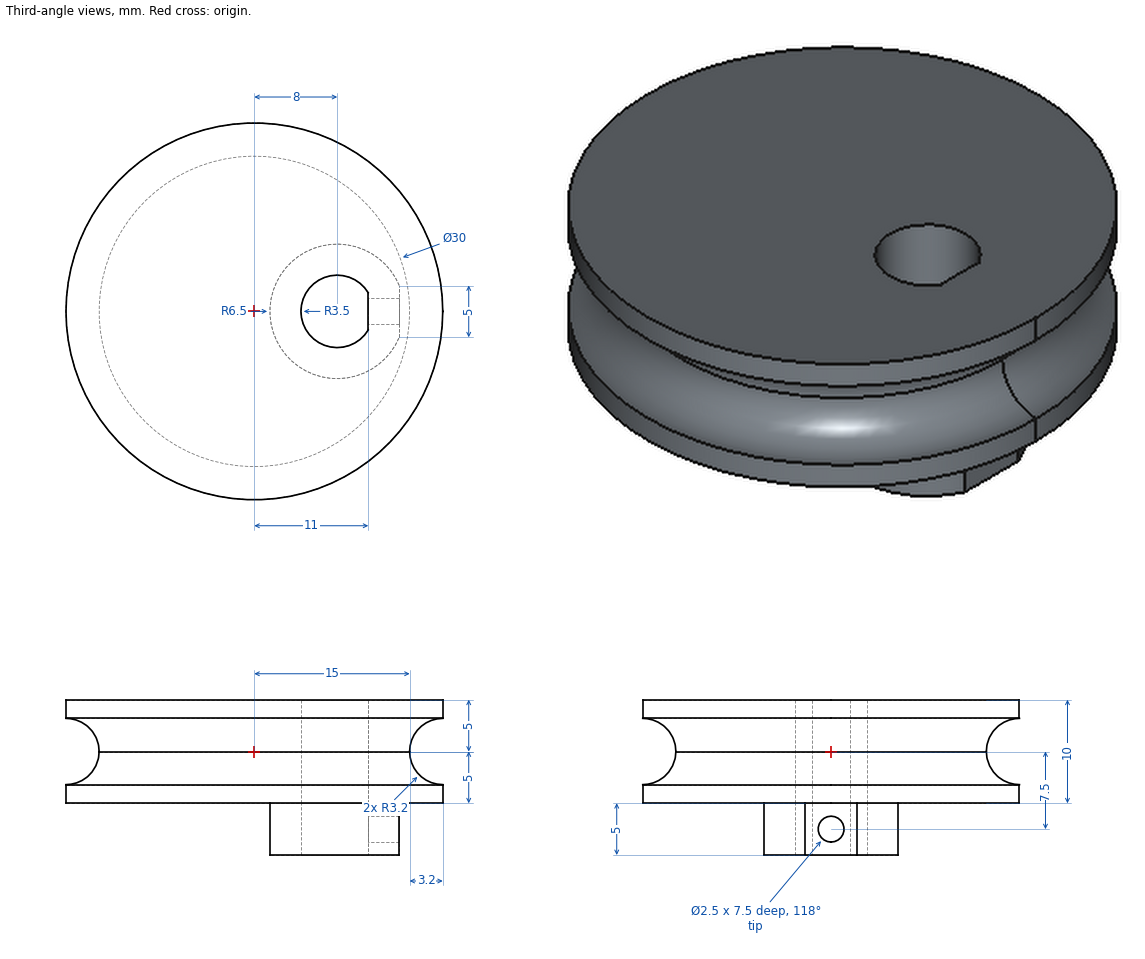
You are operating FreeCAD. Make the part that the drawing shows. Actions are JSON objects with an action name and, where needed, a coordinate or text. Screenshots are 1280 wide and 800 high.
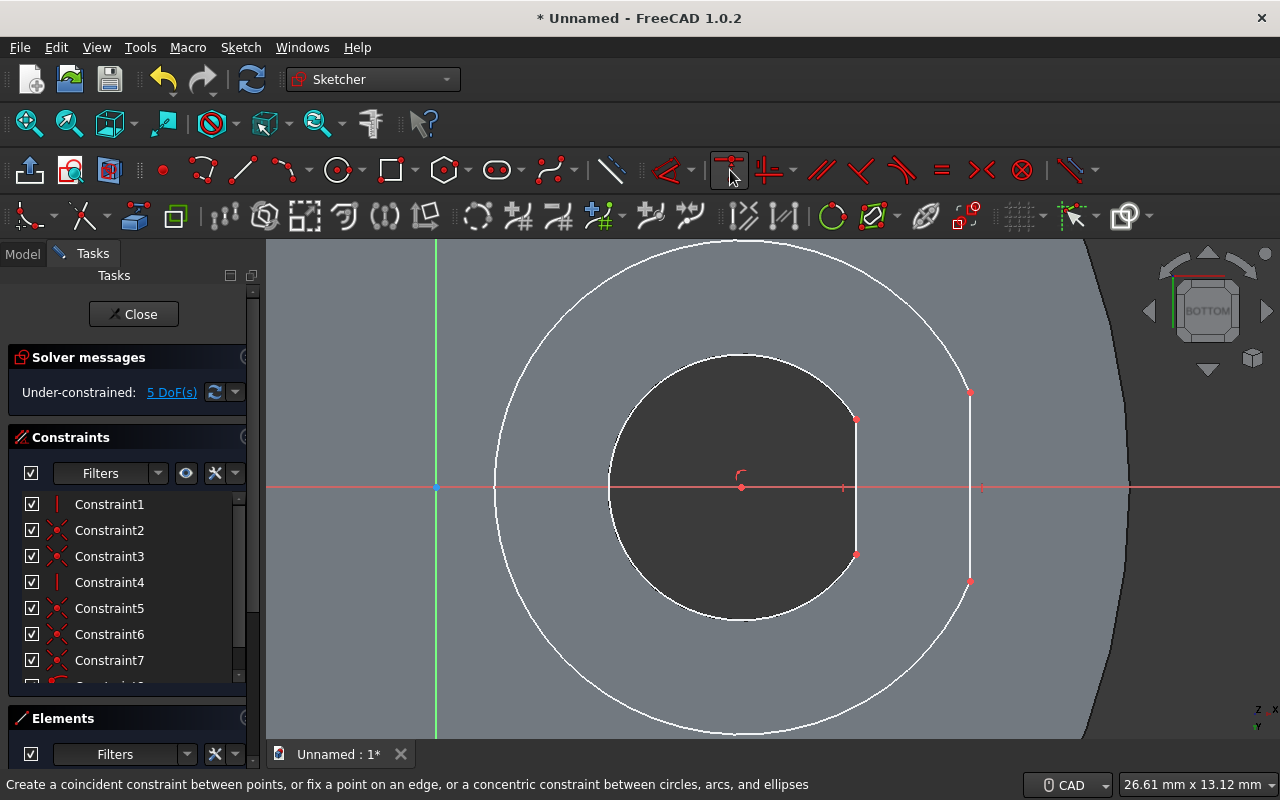
{"action": "left_click", "coordinate": [666, 170]}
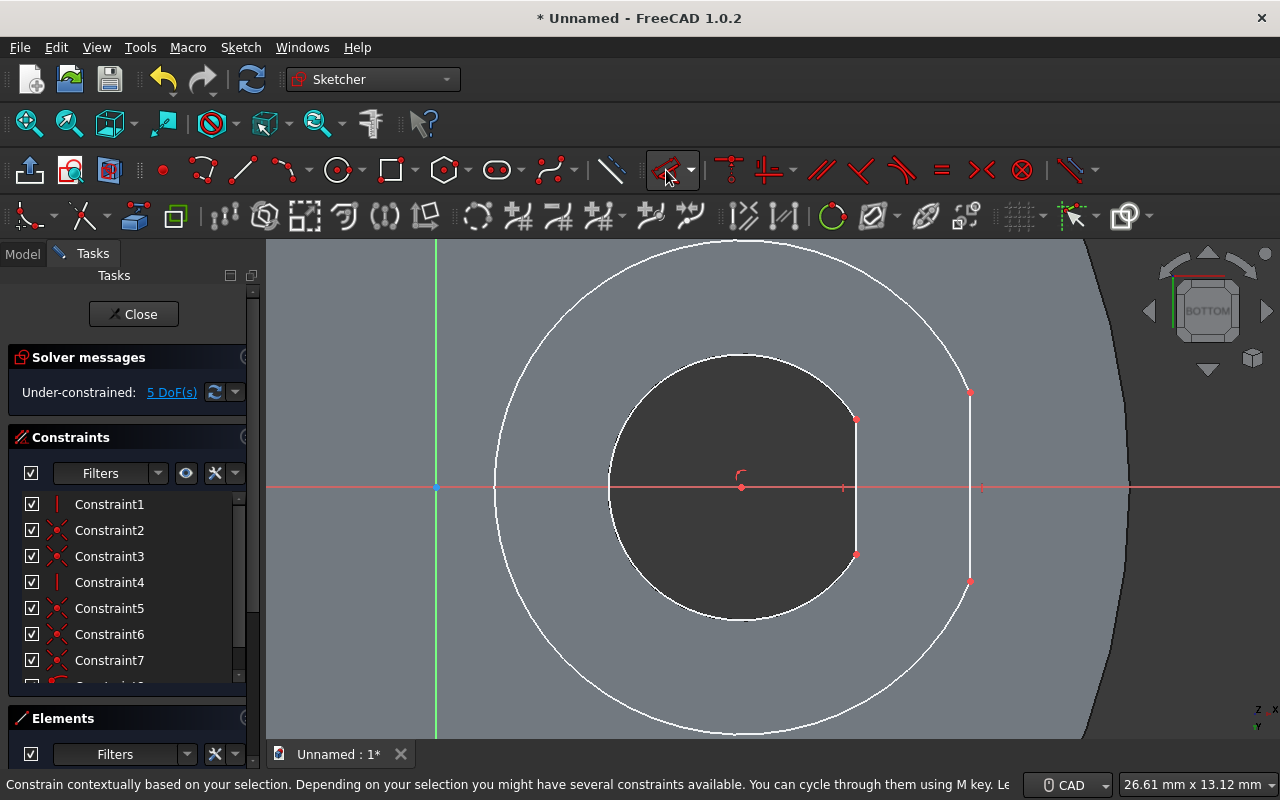
{"action": "left_click", "coordinate": [629, 267]}
{"action": "left_click", "coordinate": [511, 330]}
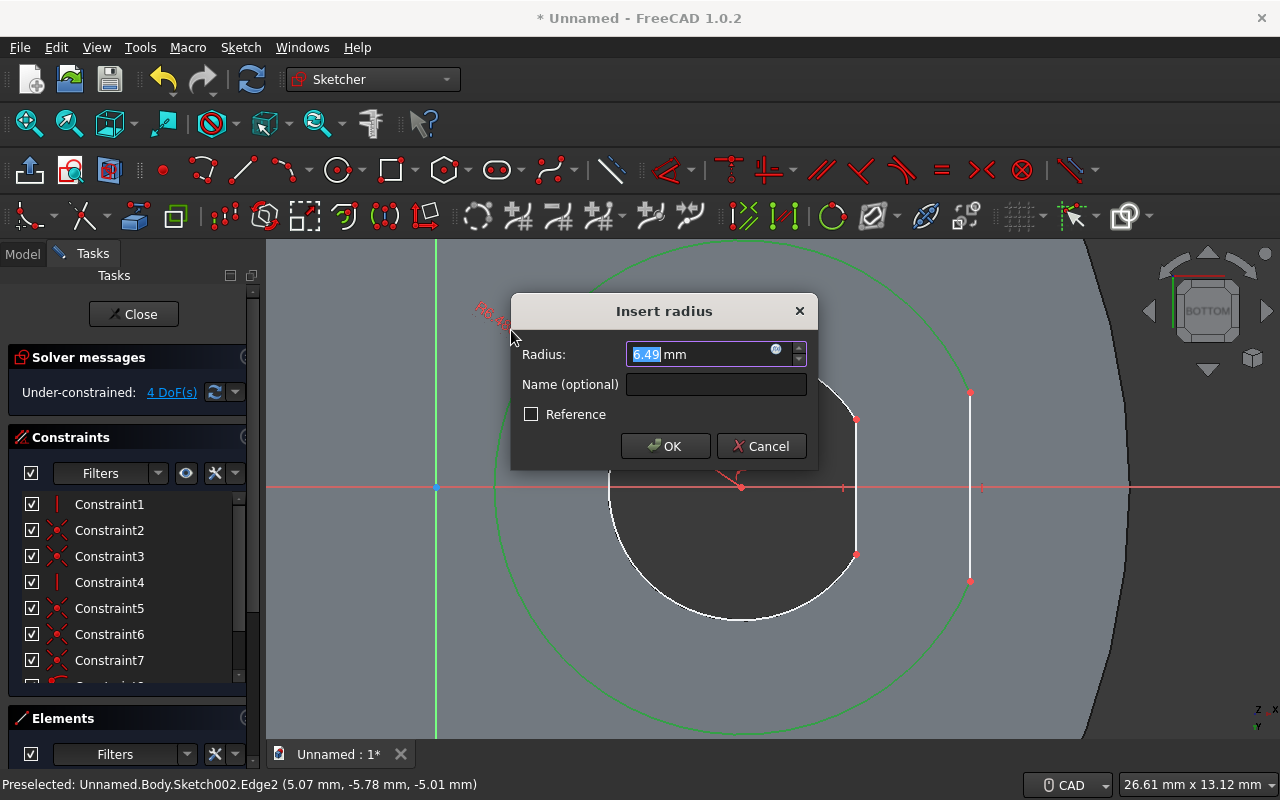
{"action": "type", "text": "6.5"}
{"action": "key", "text": "Return"}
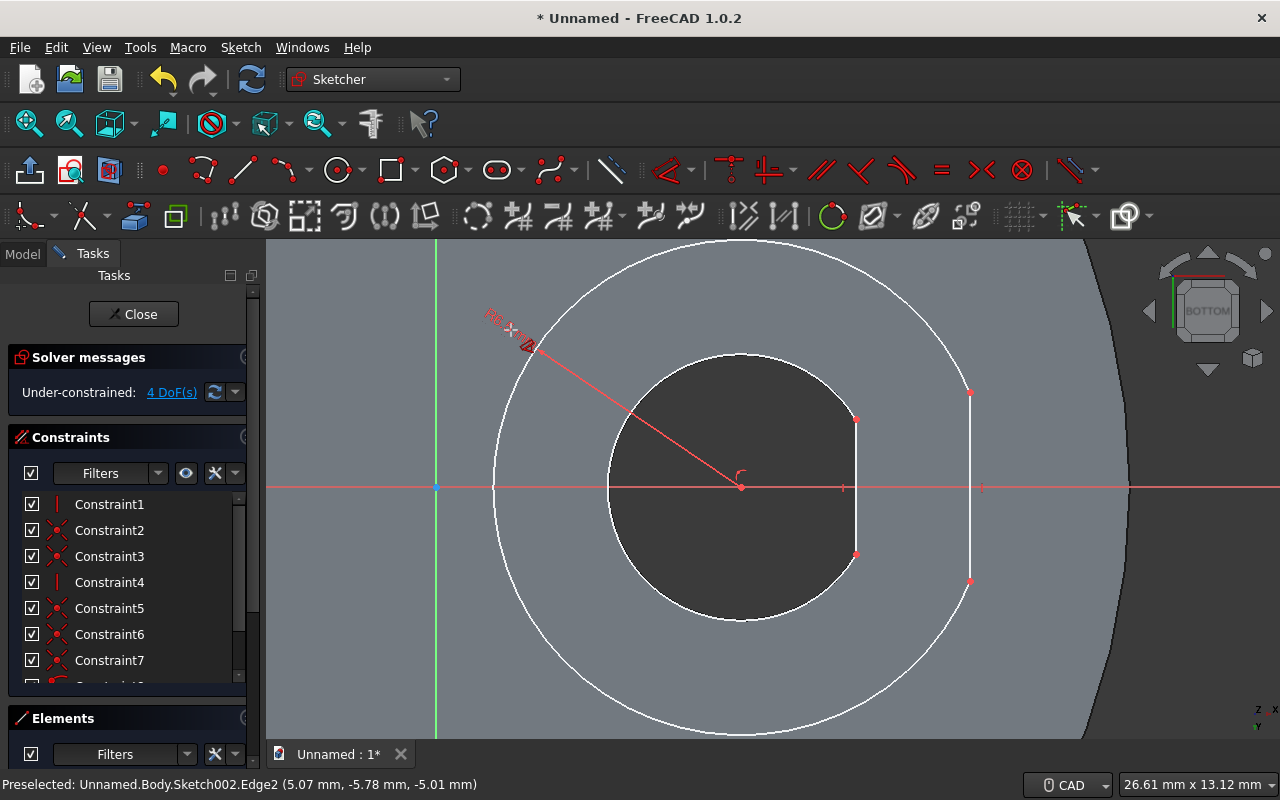
{"action": "left_click", "coordinate": [674, 372]}
{"action": "left_click", "coordinate": [658, 344]}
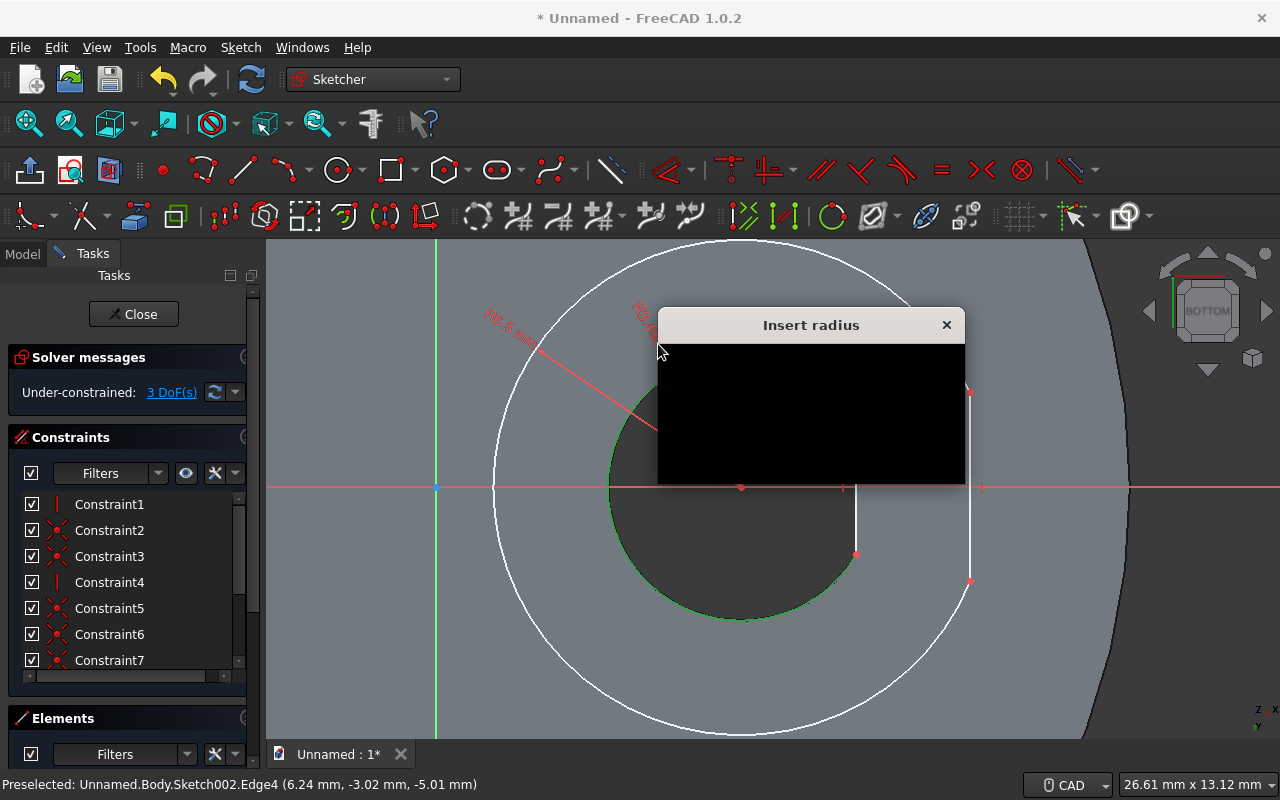
{"action": "type", "text": "3.5"}
{"action": "key", "text": "Return"}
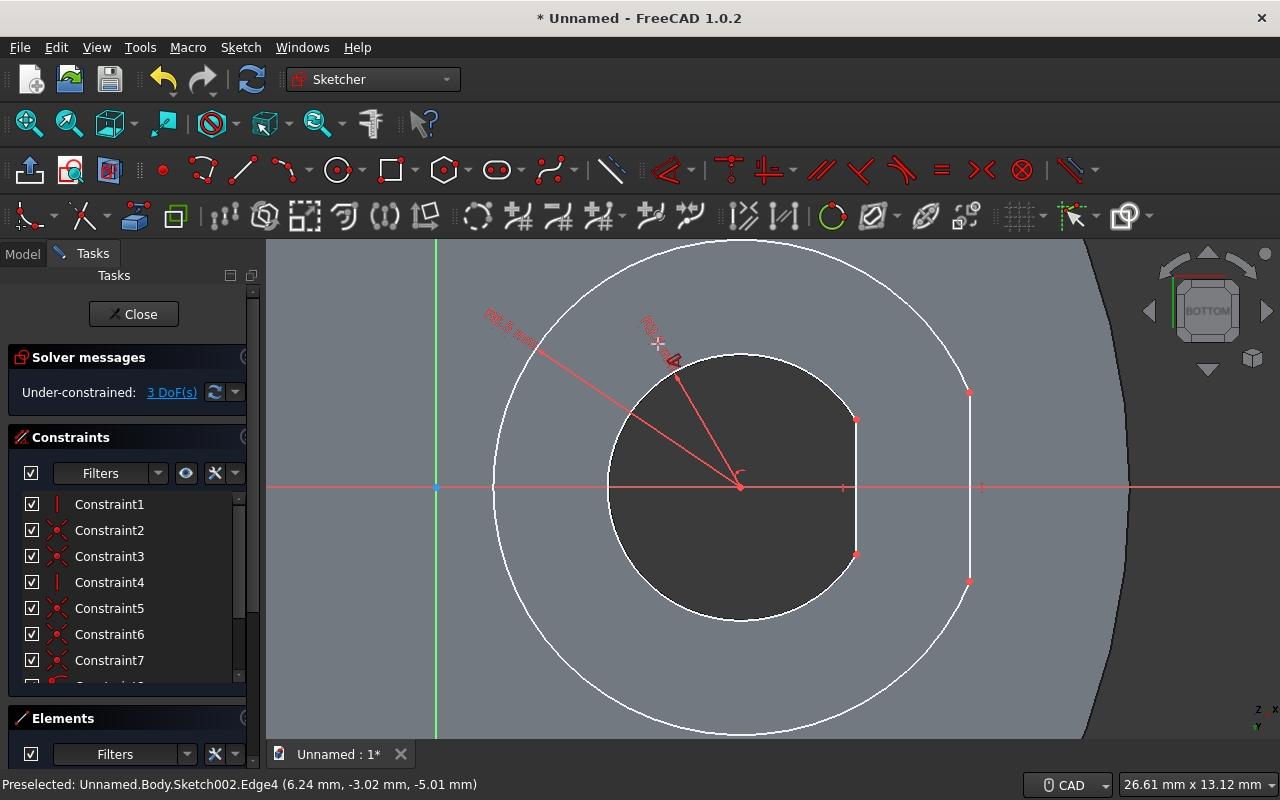
{"action": "left_click", "coordinate": [970, 450]}
{"action": "left_click", "coordinate": [1004, 444]}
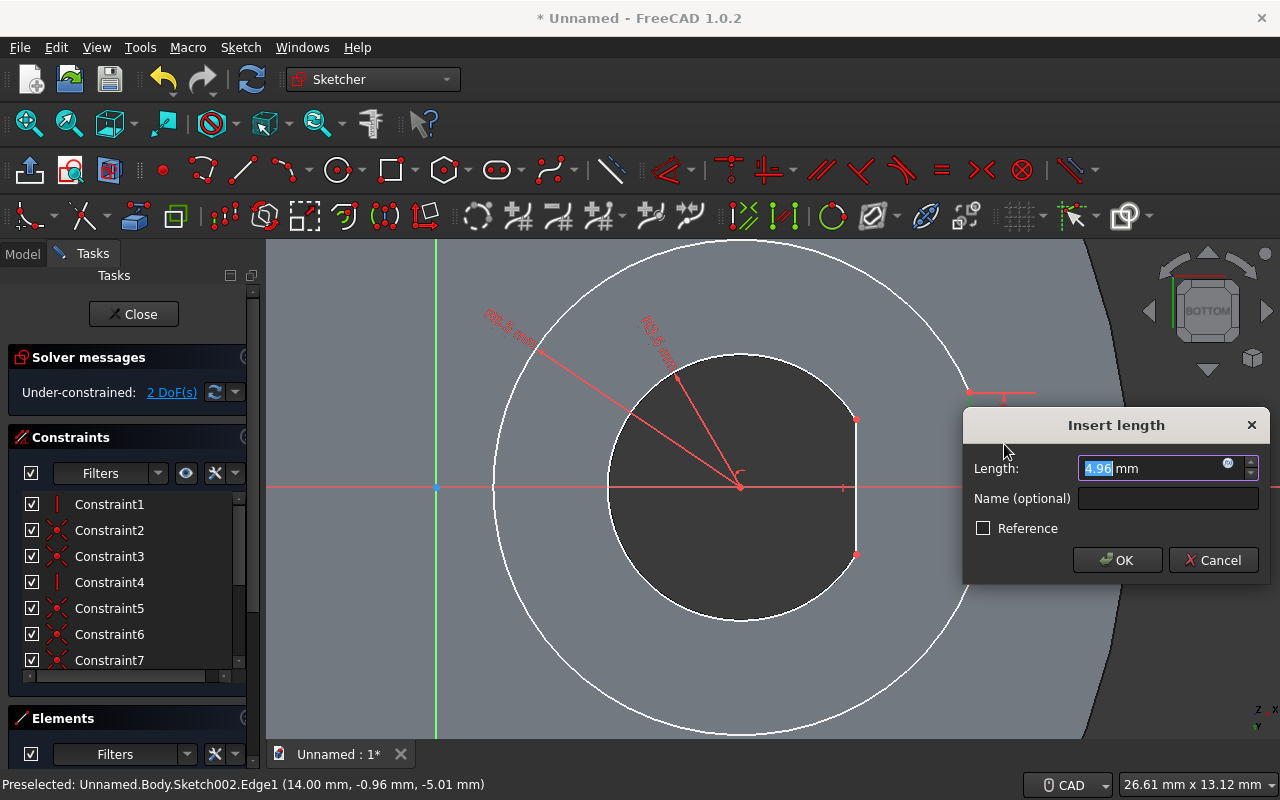
{"action": "type", "text": "5"}
{"action": "key", "text": "Return"}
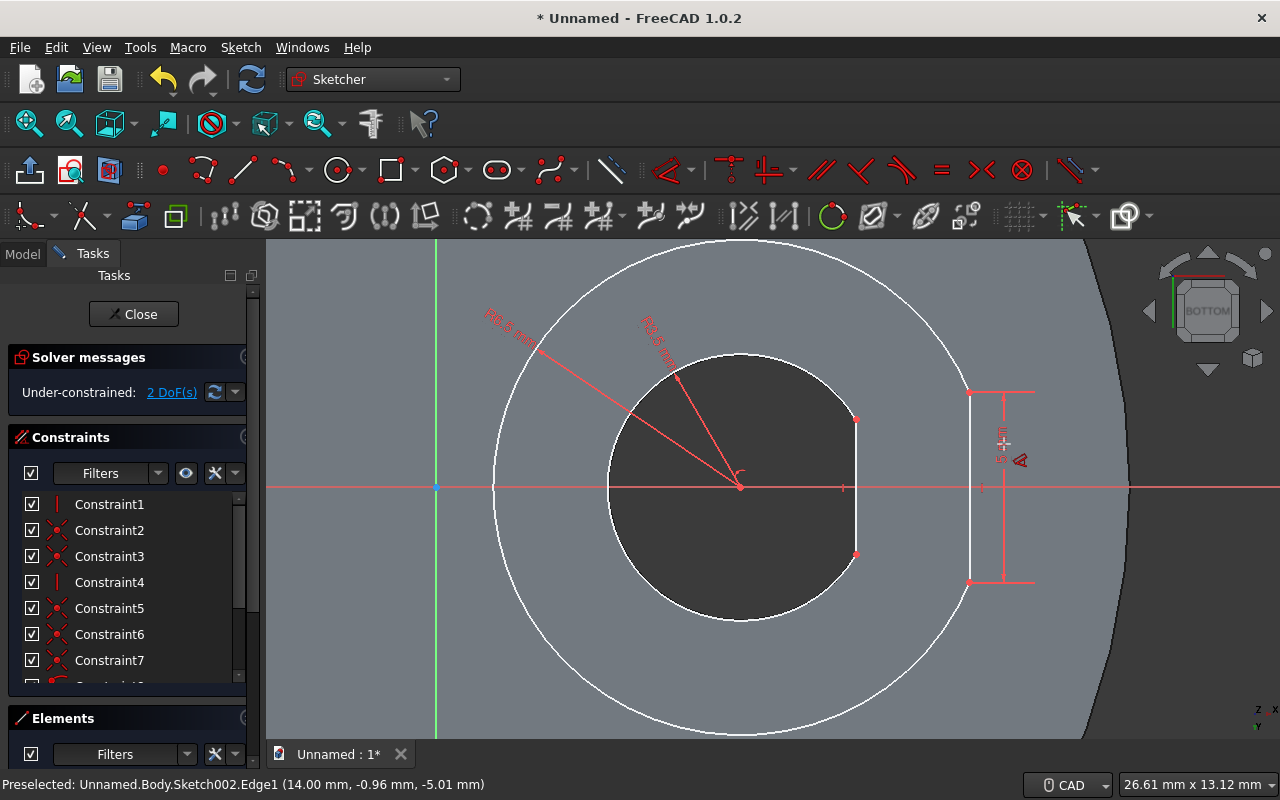
{"action": "left_click", "coordinate": [741, 487]}
{"action": "left_click", "coordinate": [589, 521]}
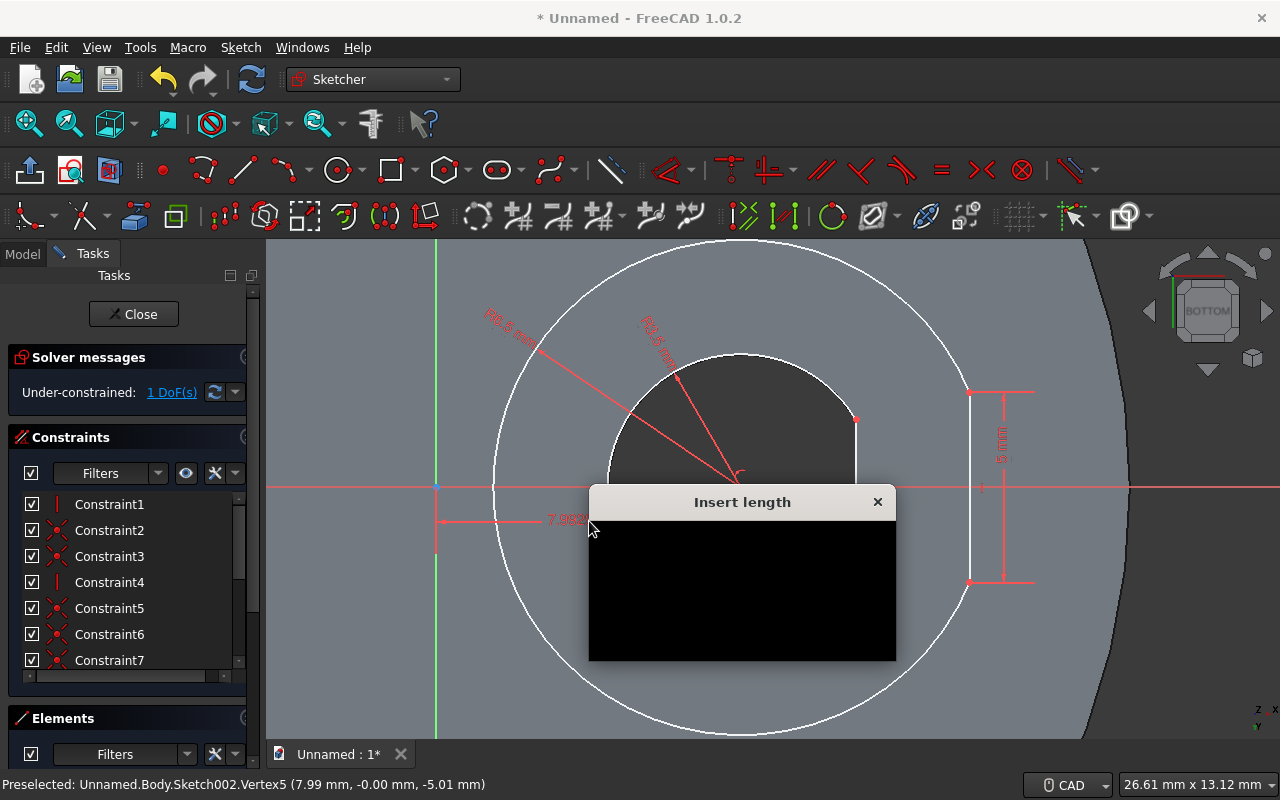
{"action": "type", "text": "8"}
{"action": "key", "text": "Return"}